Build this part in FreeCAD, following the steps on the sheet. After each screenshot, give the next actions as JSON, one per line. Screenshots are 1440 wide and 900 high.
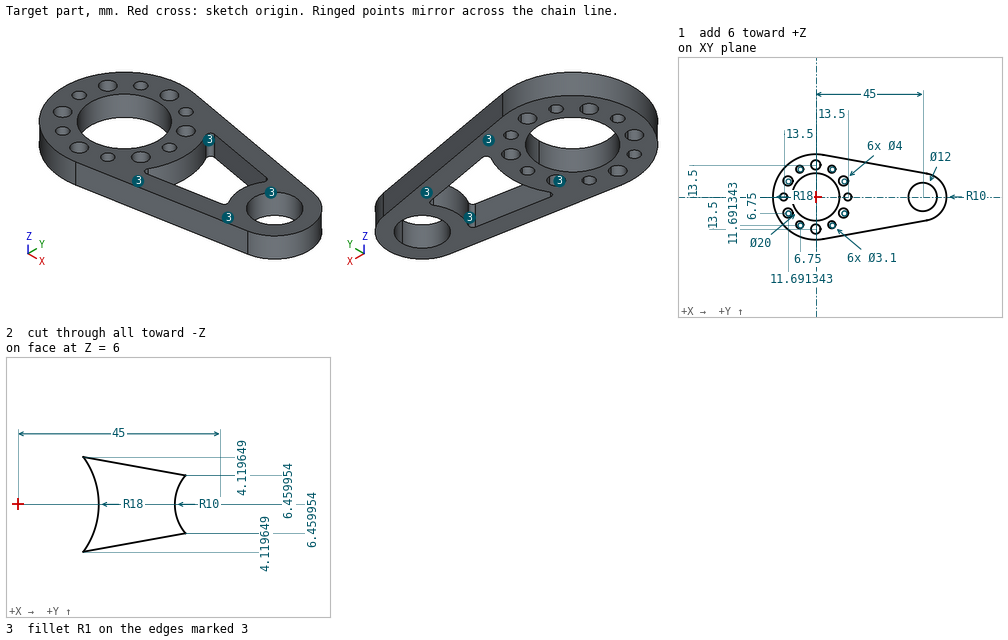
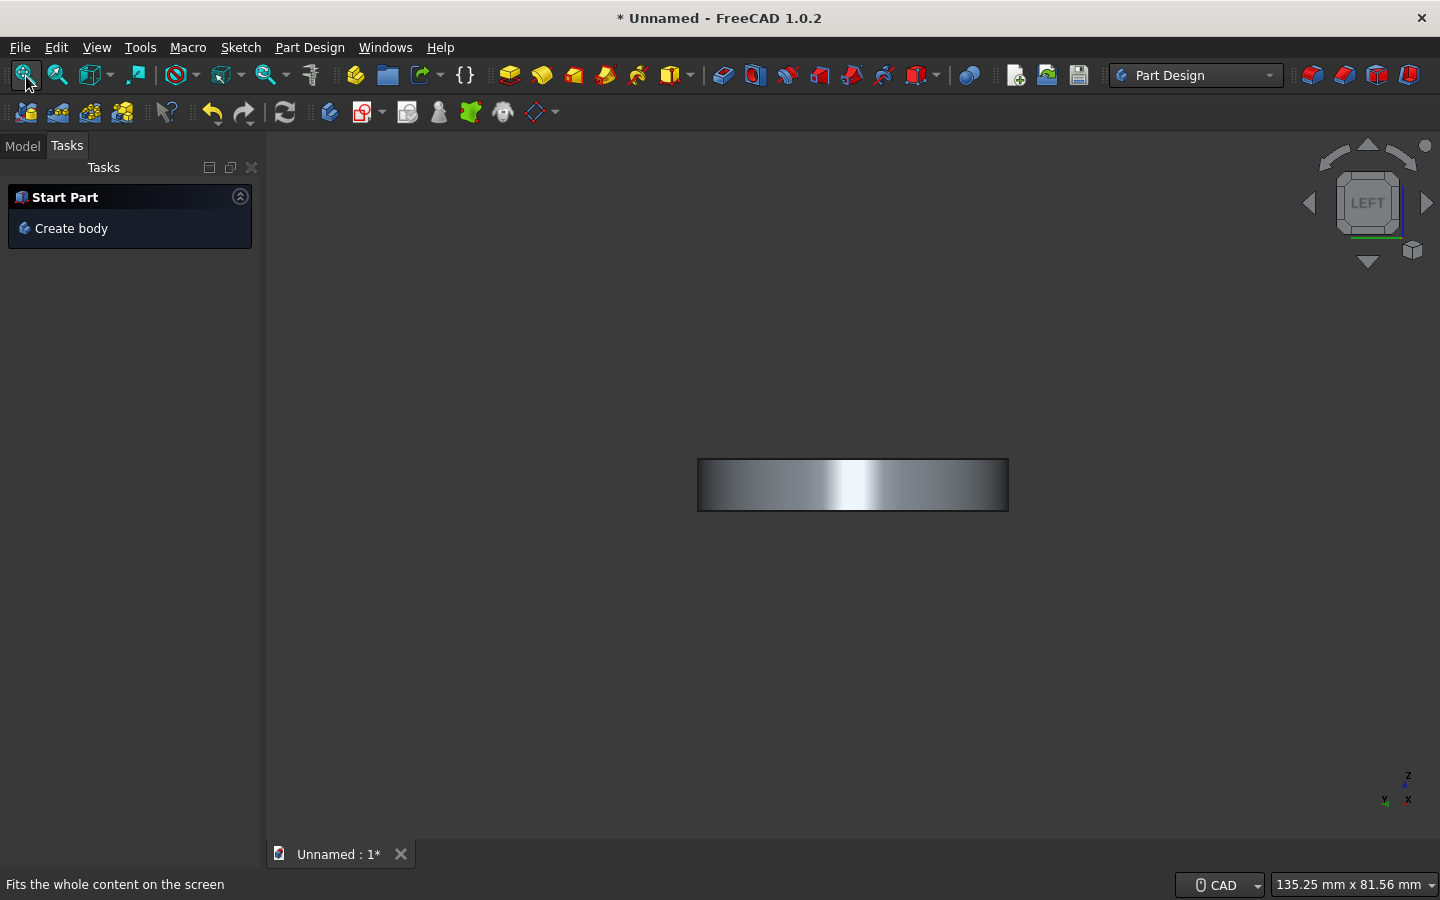
{"action": "key", "text": "v 3"}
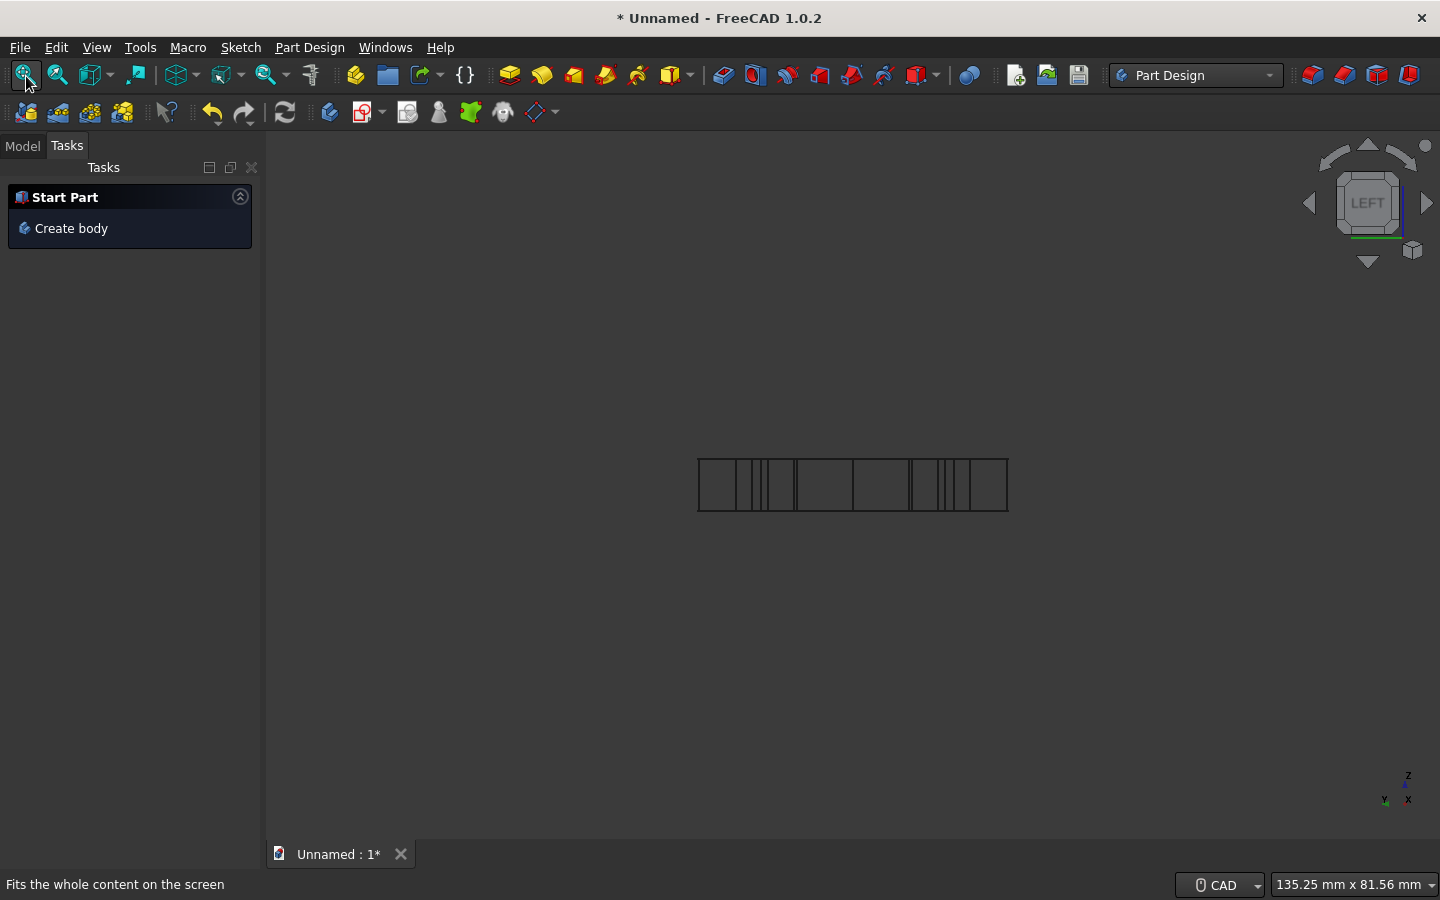
{"action": "key", "text": "0"}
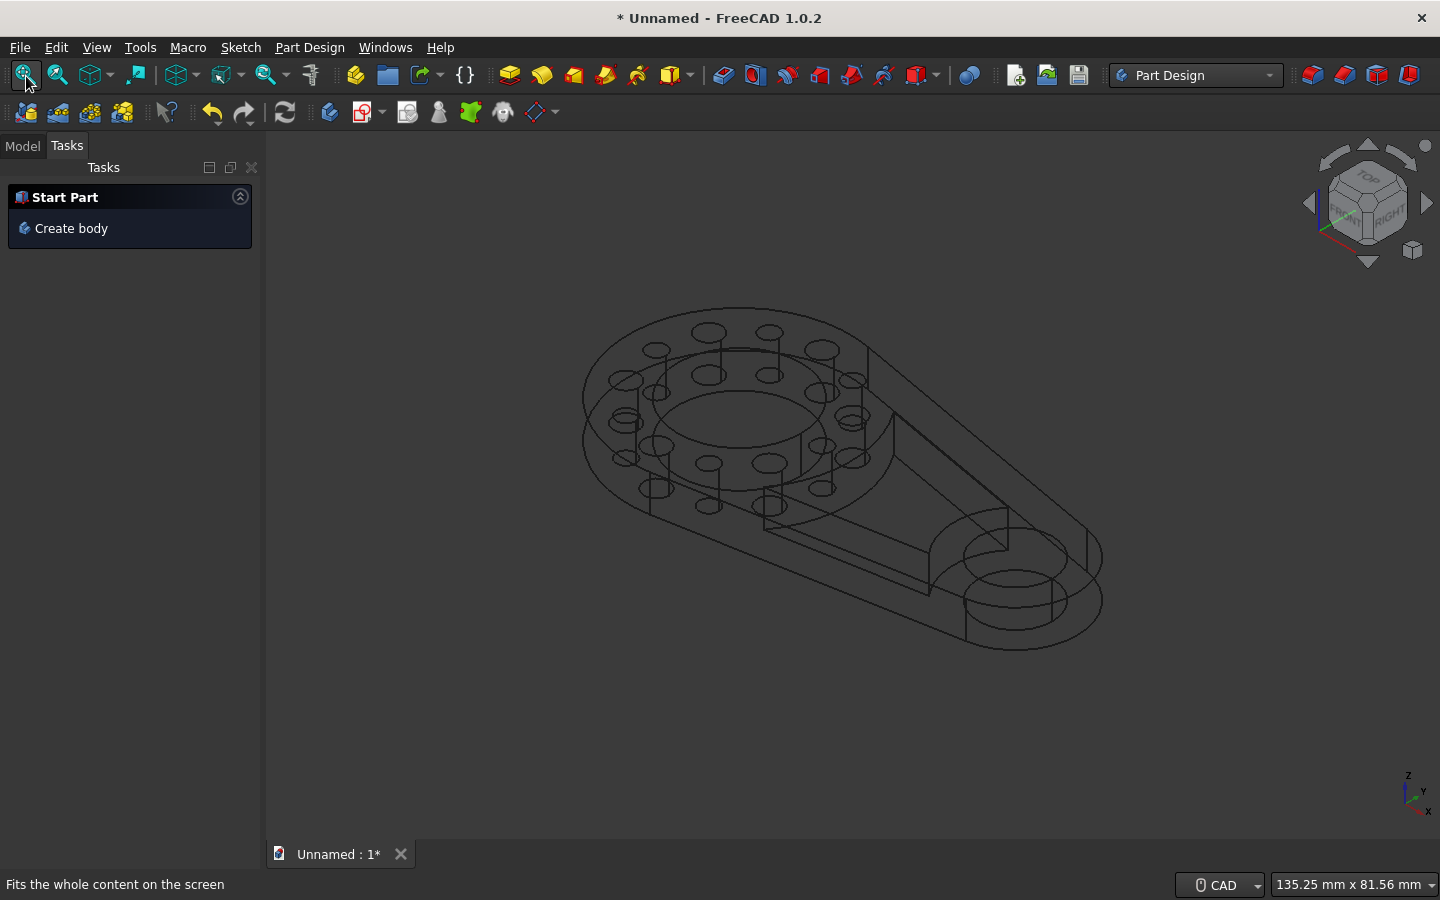
{"action": "left_click", "coordinate": [764, 507]}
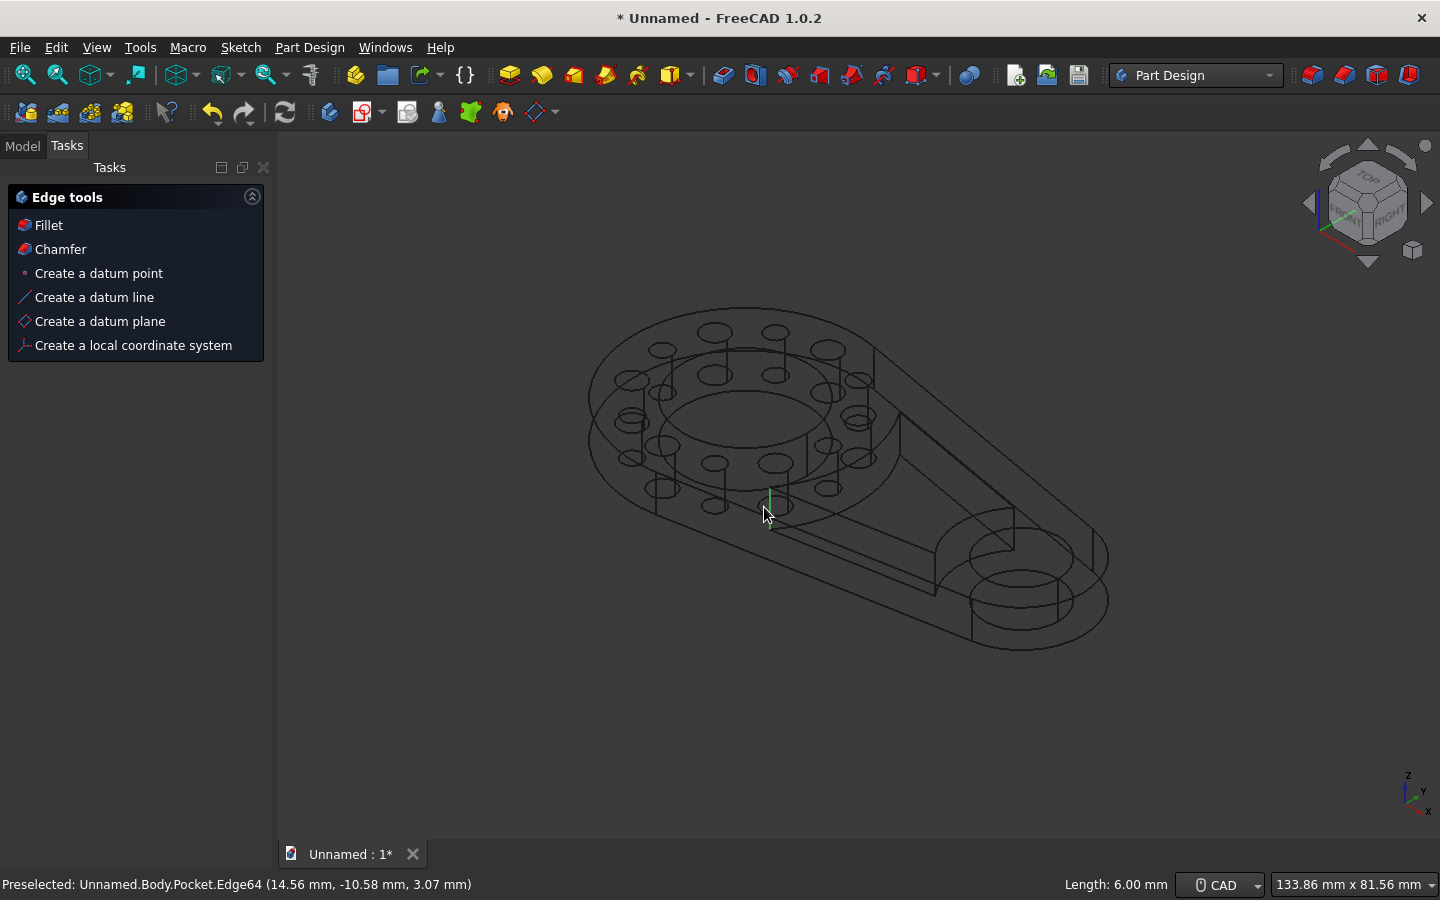
{"action": "left_click", "coordinate": [900, 432], "text": "ctrl"}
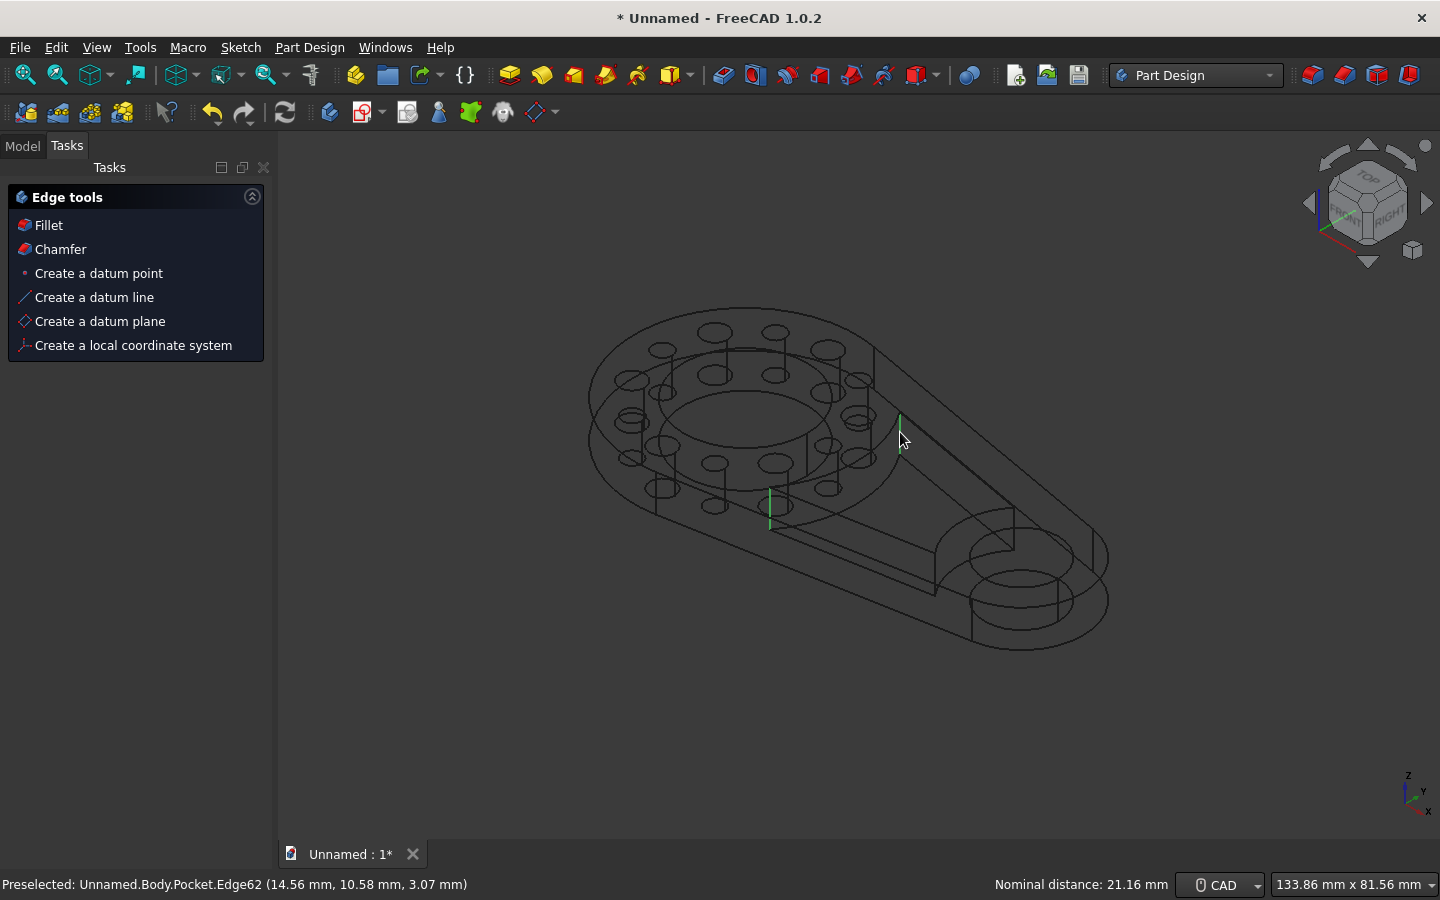
{"action": "left_click", "coordinate": [1014, 519], "text": "ctrl"}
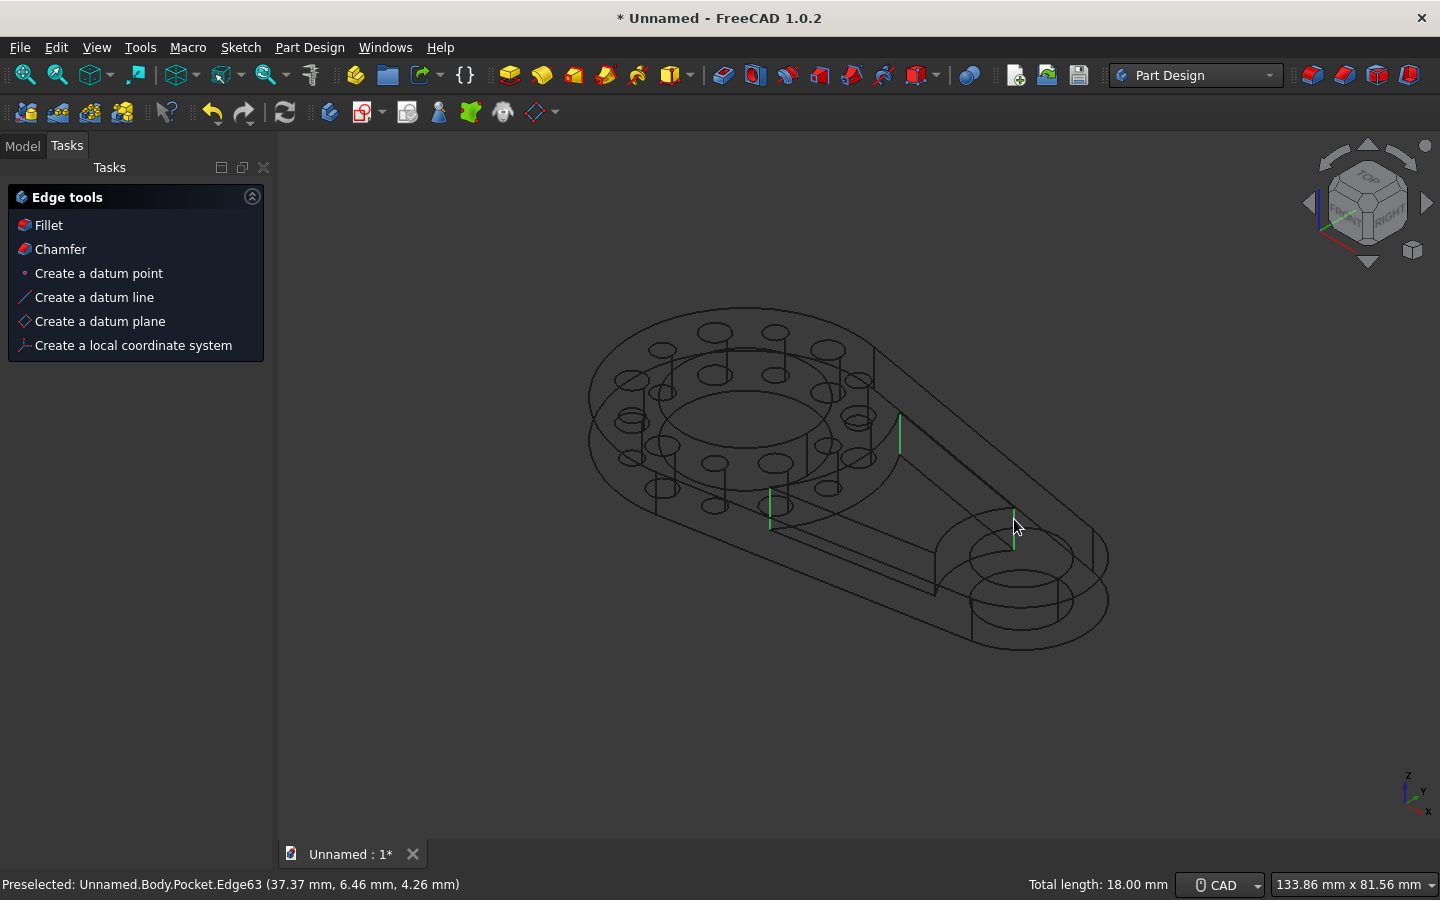
{"action": "left_click", "coordinate": [935, 574], "text": "ctrl"}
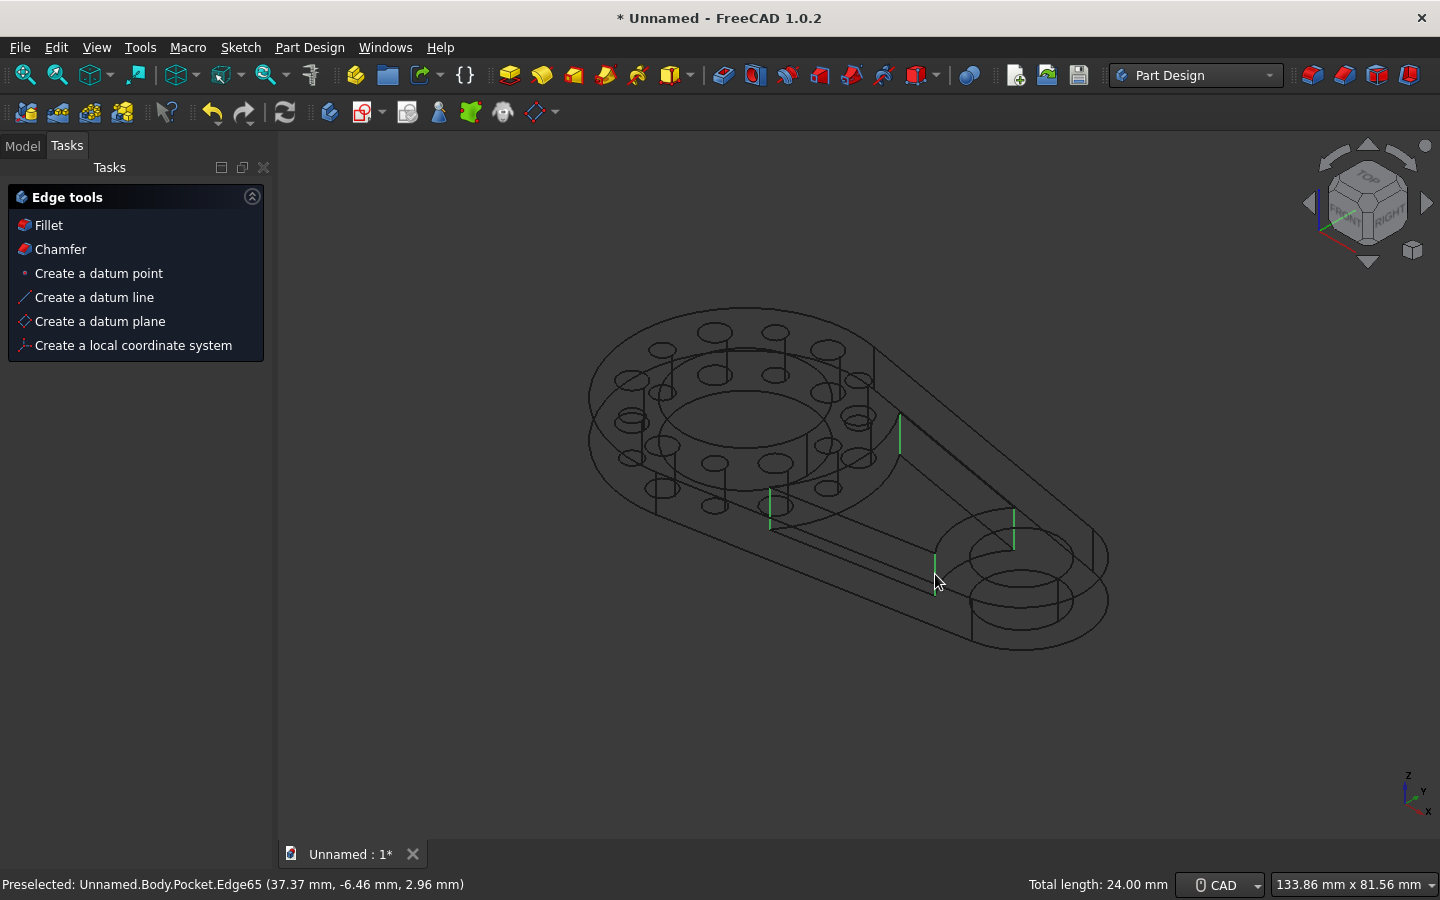
{"action": "key", "text": "v 1"}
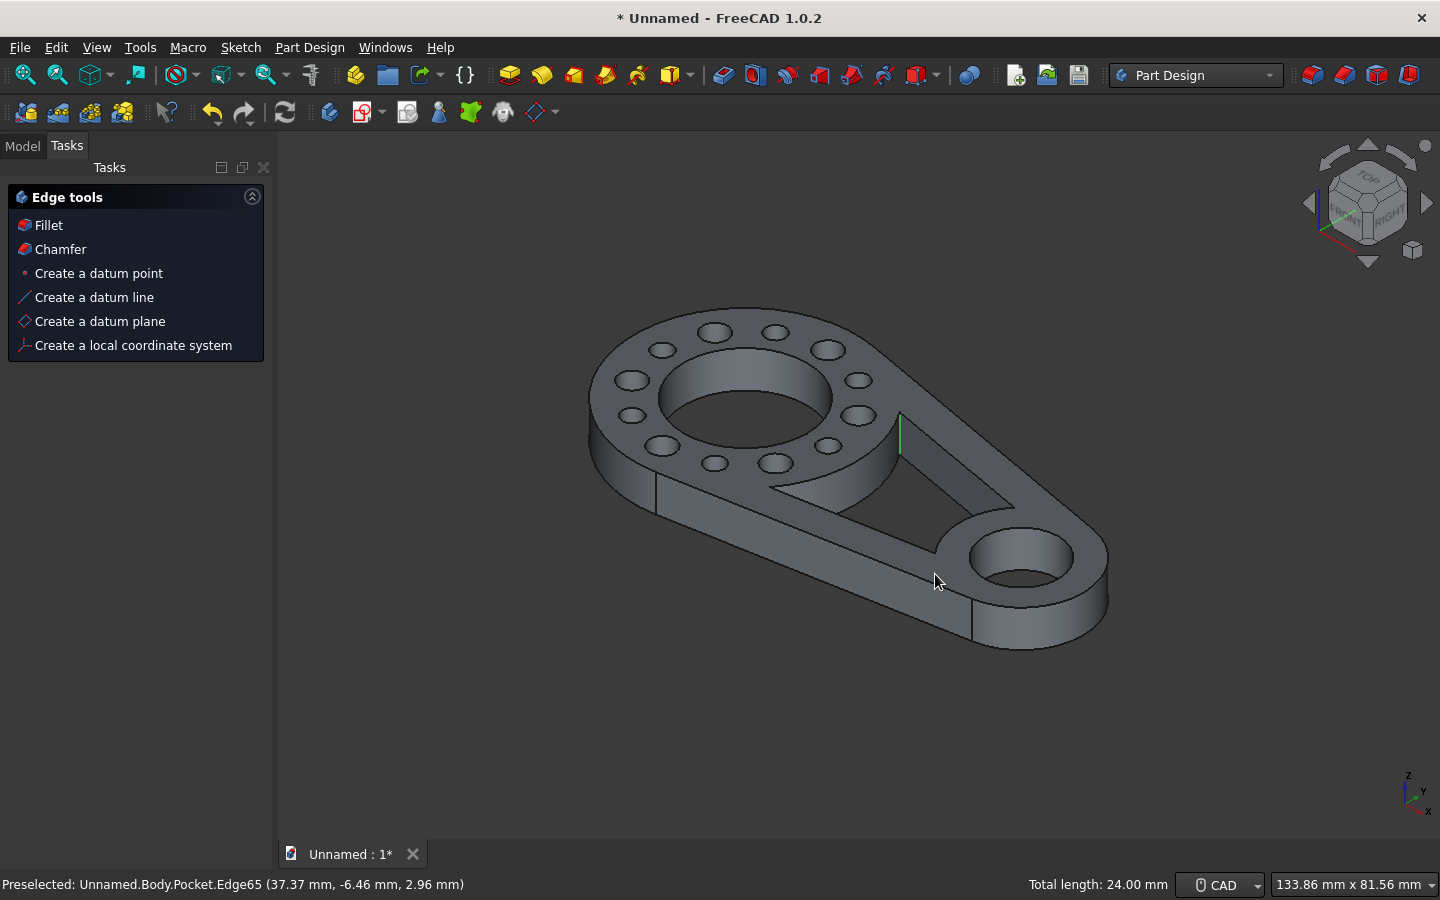
{"action": "left_click", "coordinate": [1314, 76]}